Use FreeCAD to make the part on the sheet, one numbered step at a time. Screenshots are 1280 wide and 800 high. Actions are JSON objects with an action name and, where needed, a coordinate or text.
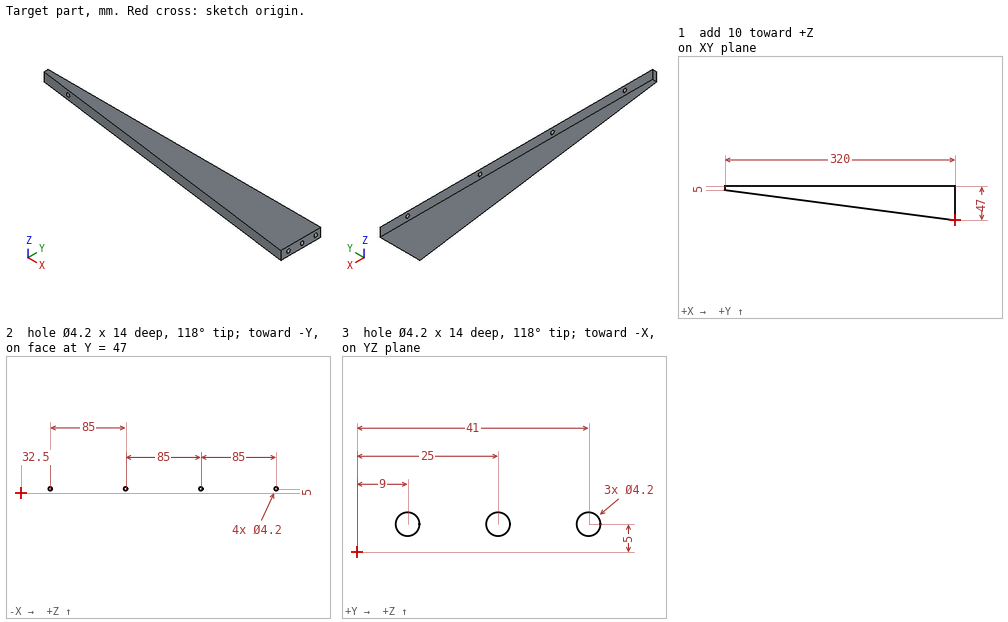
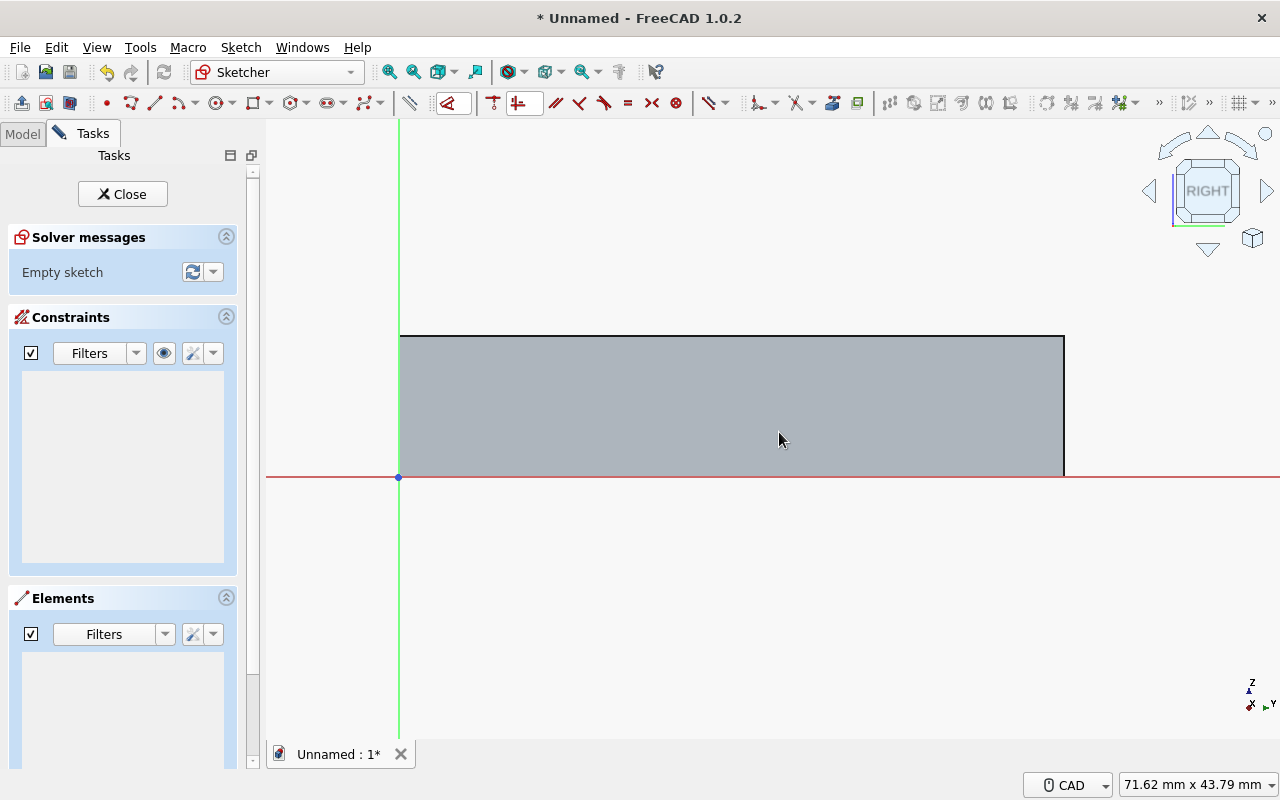
{"action": "key", "text": "g c"}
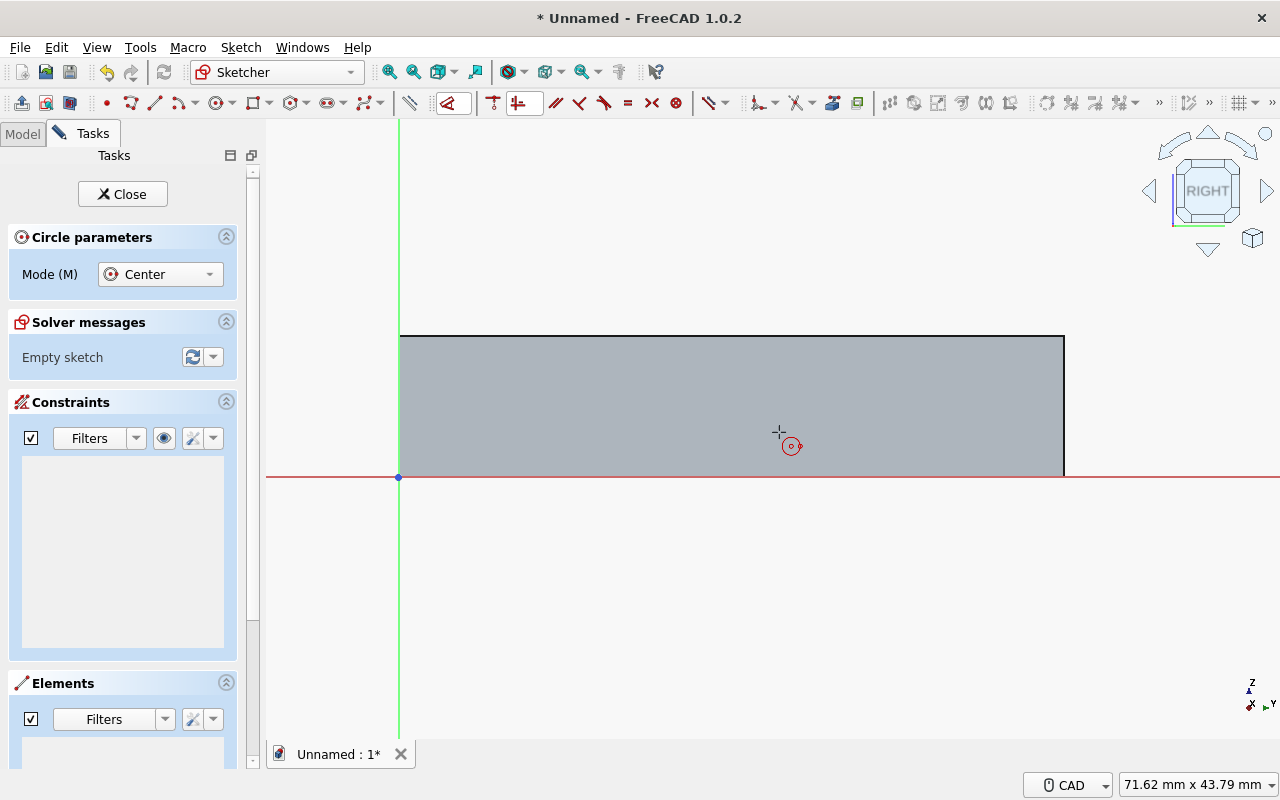
{"action": "left_click", "coordinate": [979, 407]}
{"action": "mouse_move", "coordinate": [1000, 386]}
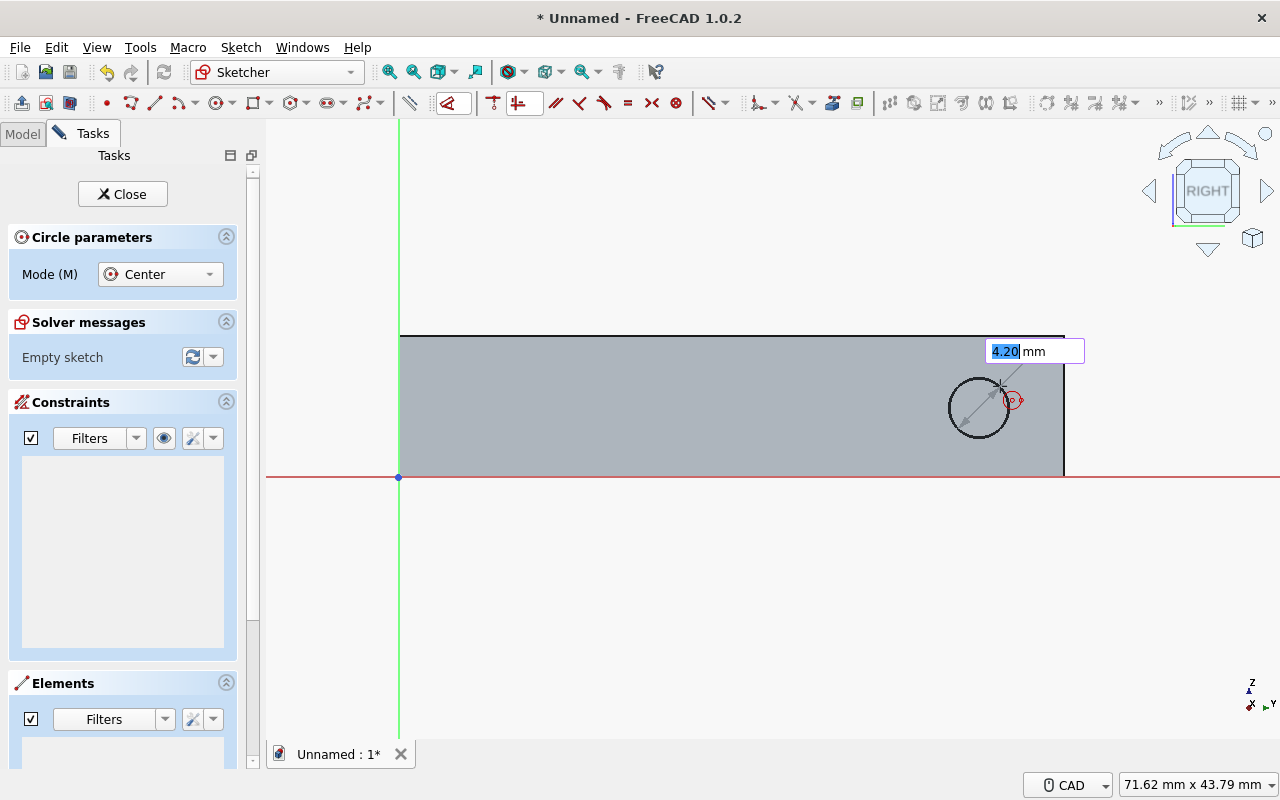
{"action": "type", "text": "4.2"}
{"action": "key", "text": "Return"}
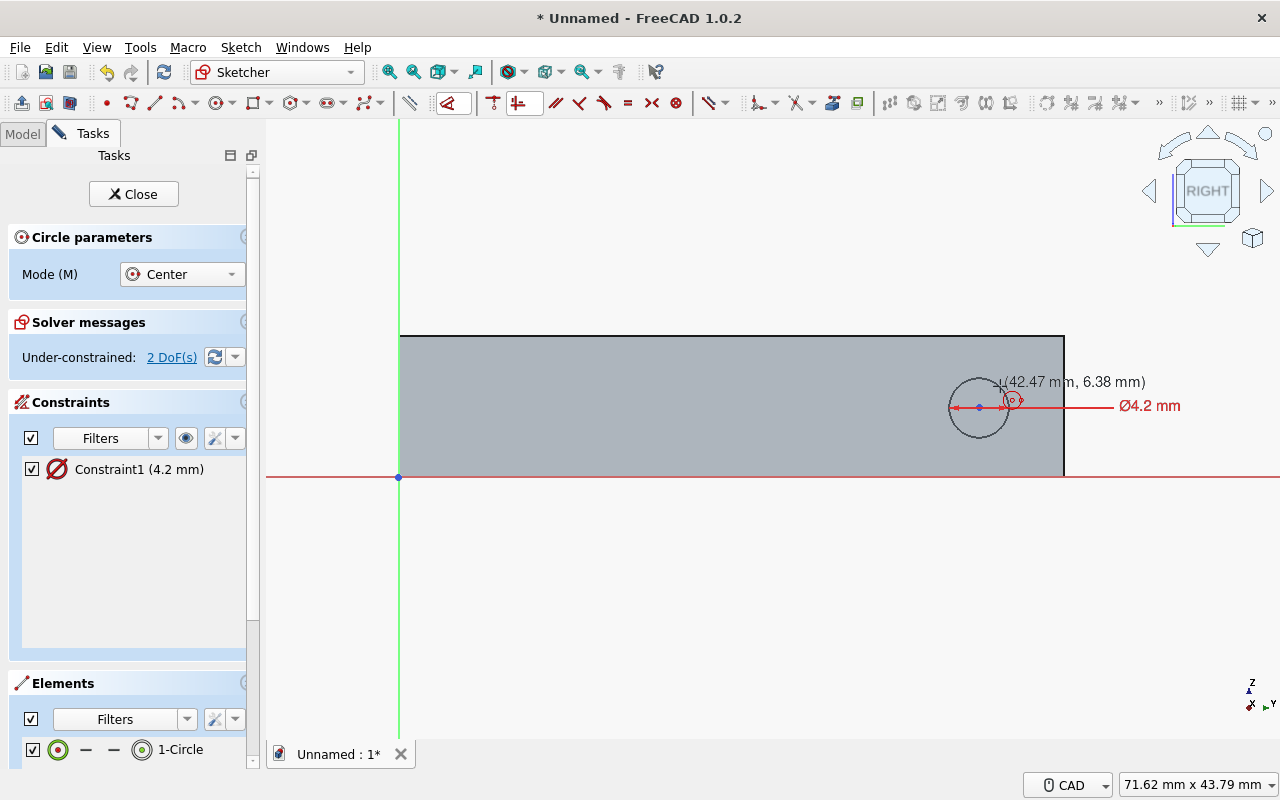
{"action": "left_click", "coordinate": [753, 407]}
{"action": "mouse_move", "coordinate": [774, 386]}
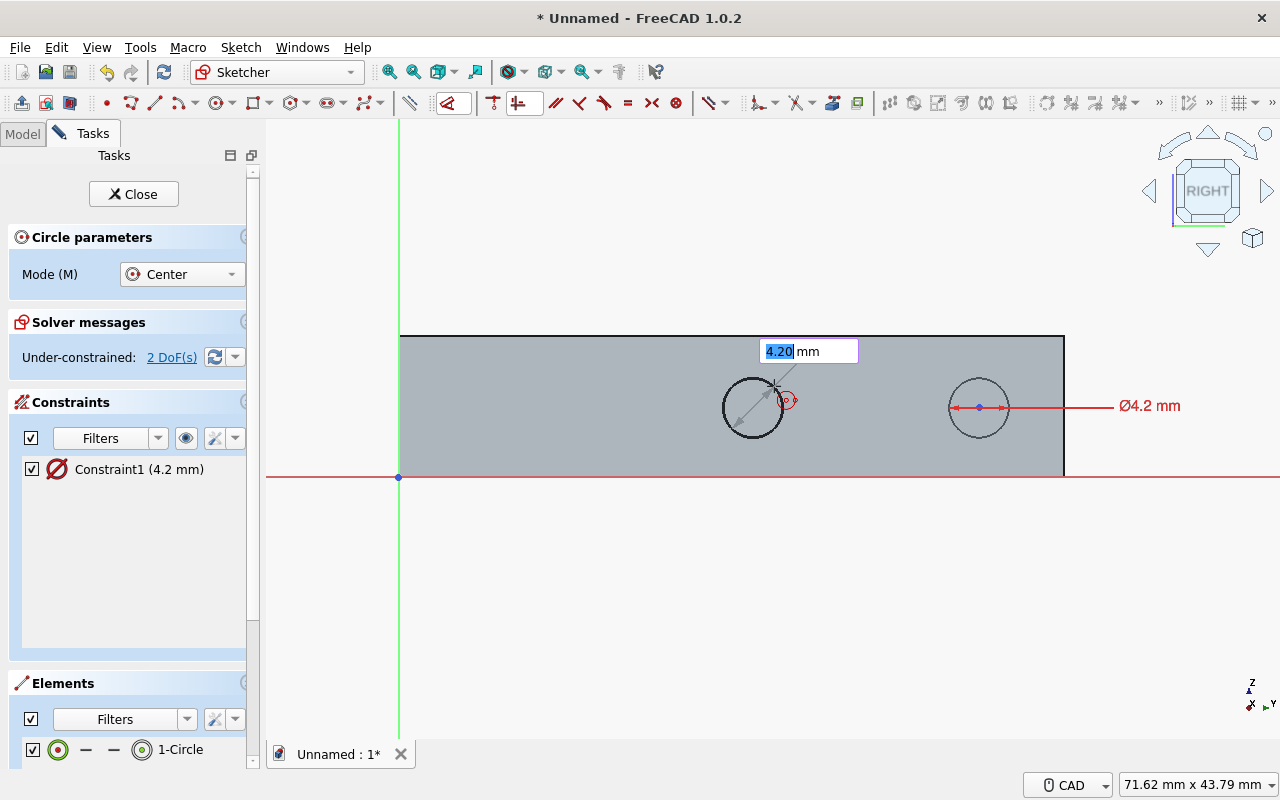
{"action": "type", "text": "4.2"}
{"action": "key", "text": "Return"}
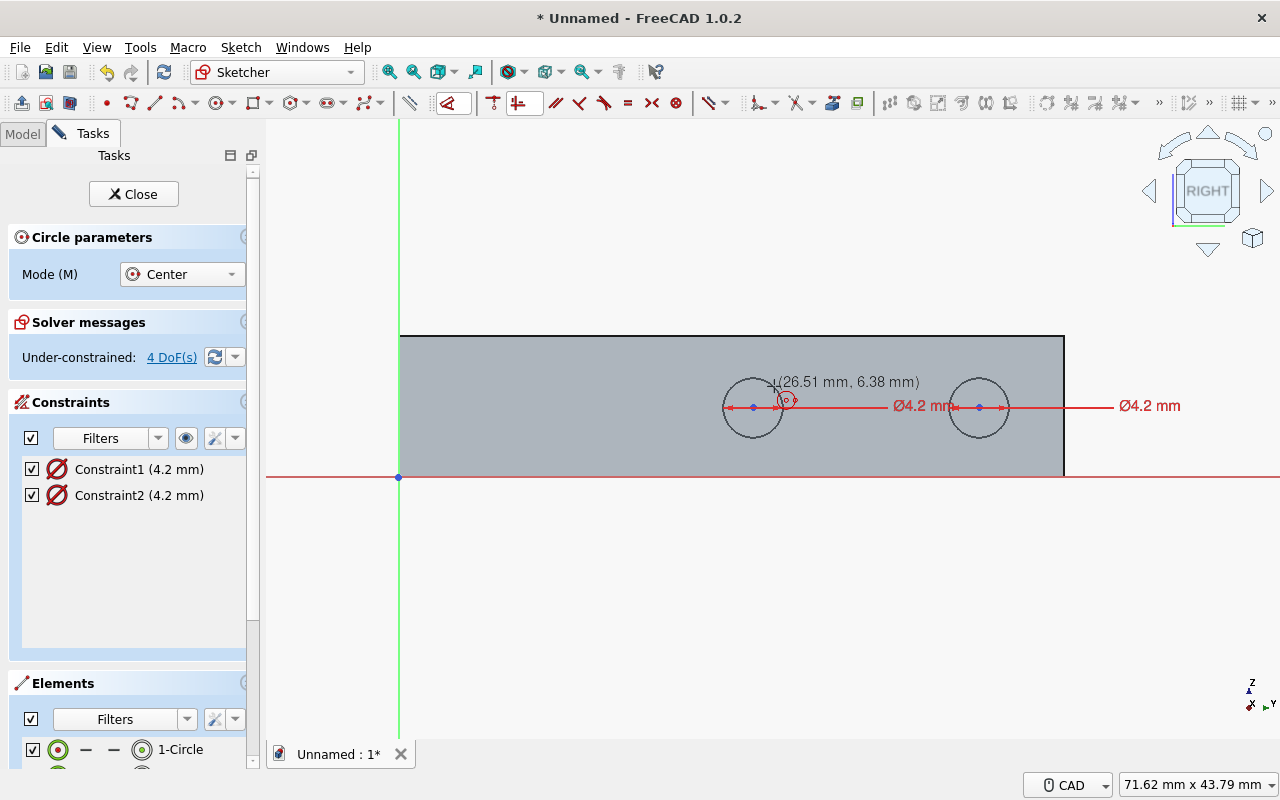
{"action": "left_click", "coordinate": [526, 407]}
{"action": "mouse_move", "coordinate": [547, 386]}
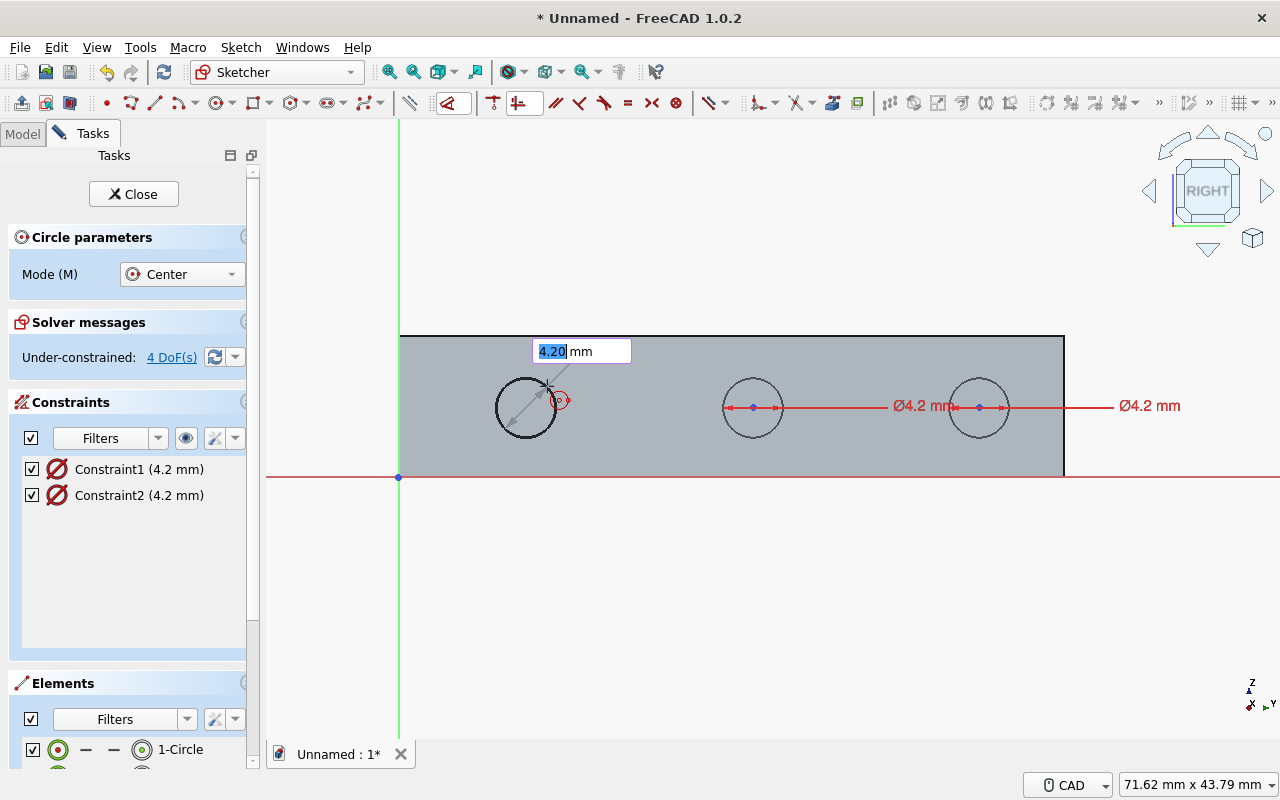
{"action": "type", "text": "4.2"}
{"action": "key", "text": "Return"}
{"action": "key", "text": "Escape"}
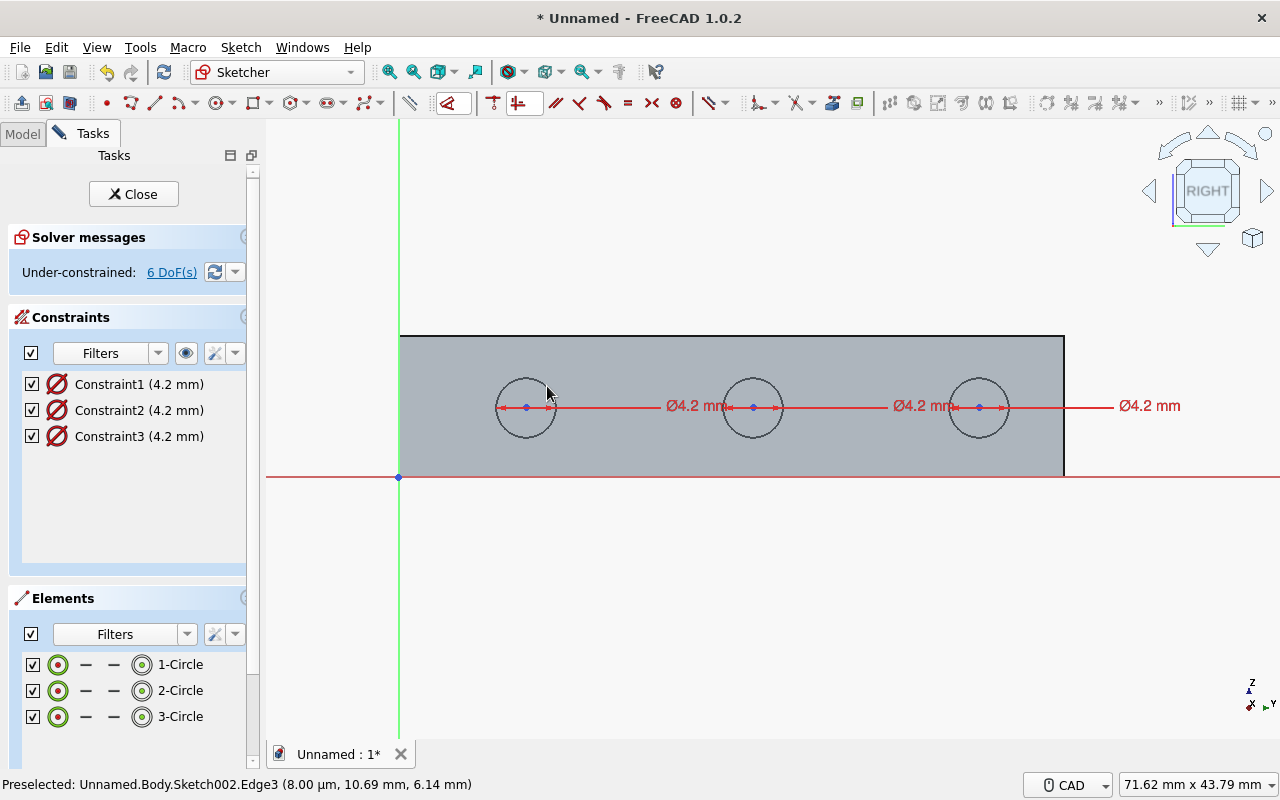
{"action": "left_click", "coordinate": [979, 408]}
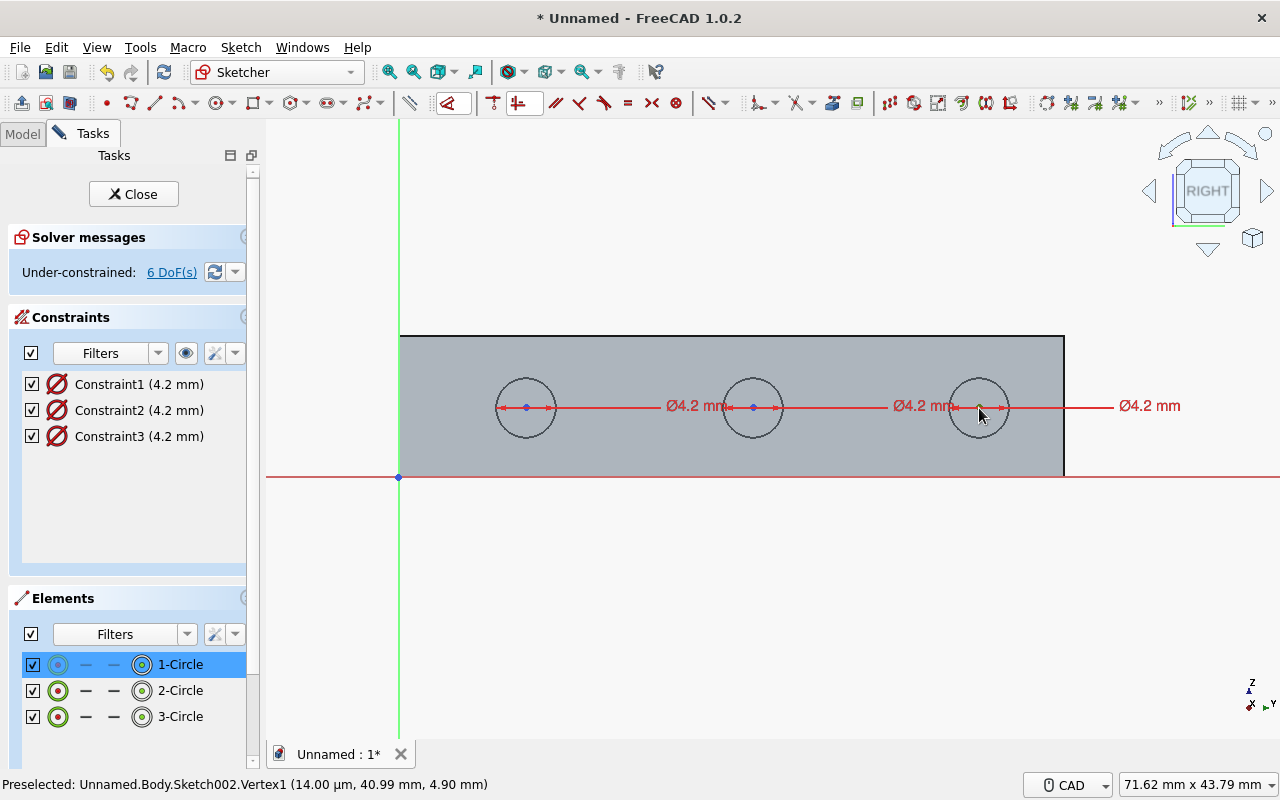
{"action": "left_click", "coordinate": [753, 408]}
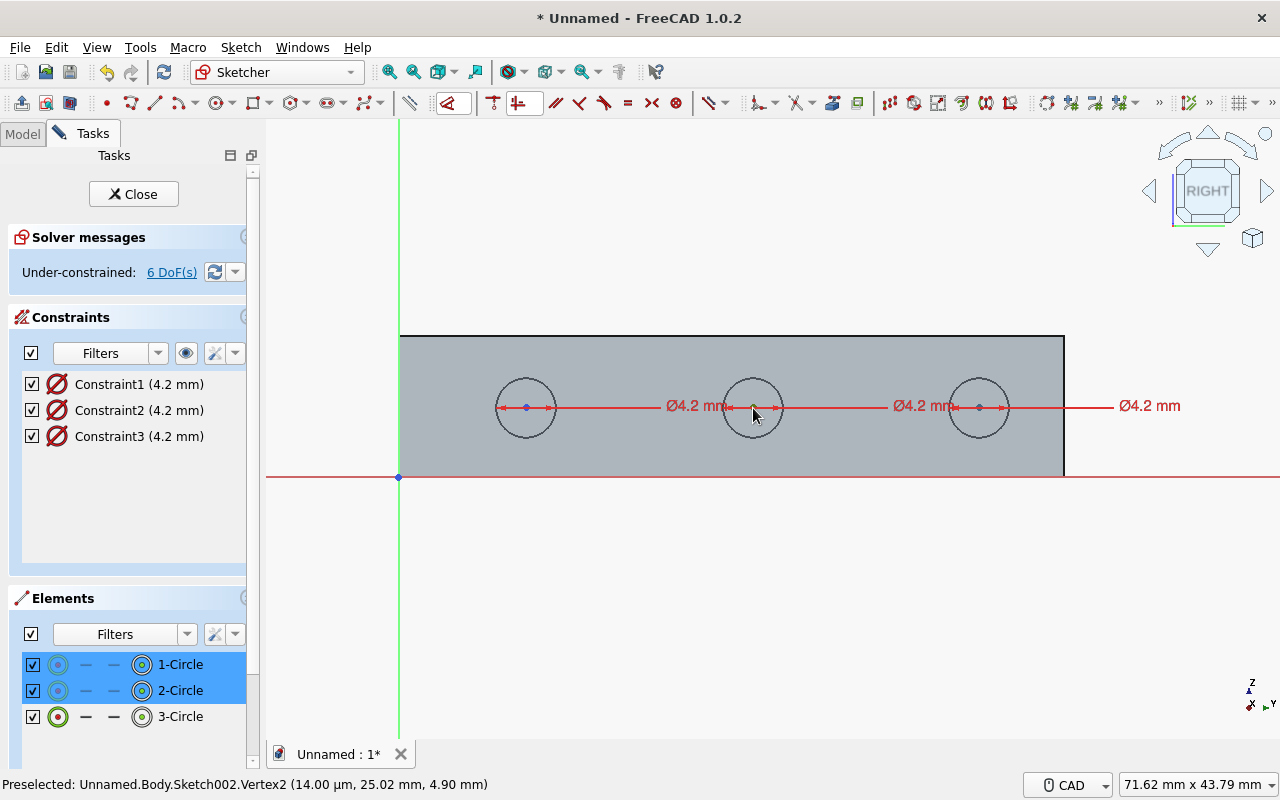
{"action": "left_click", "coordinate": [538, 104]}